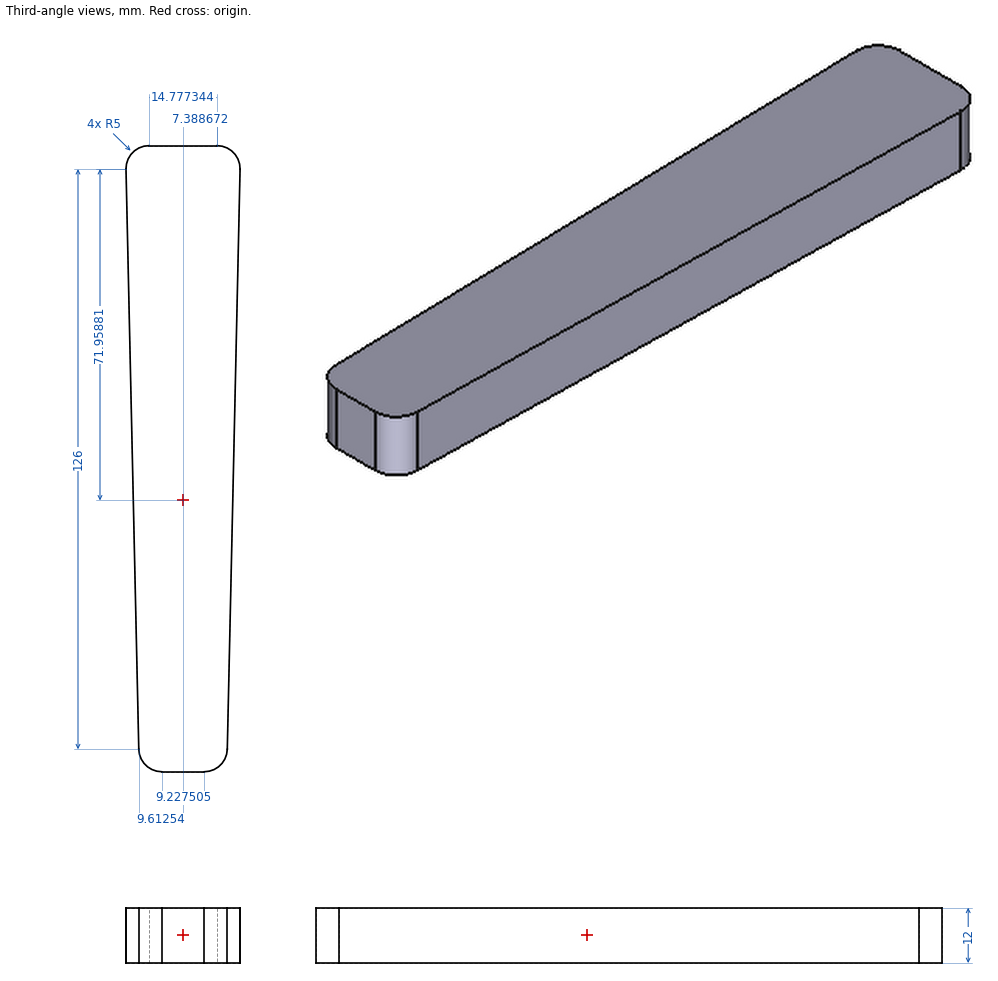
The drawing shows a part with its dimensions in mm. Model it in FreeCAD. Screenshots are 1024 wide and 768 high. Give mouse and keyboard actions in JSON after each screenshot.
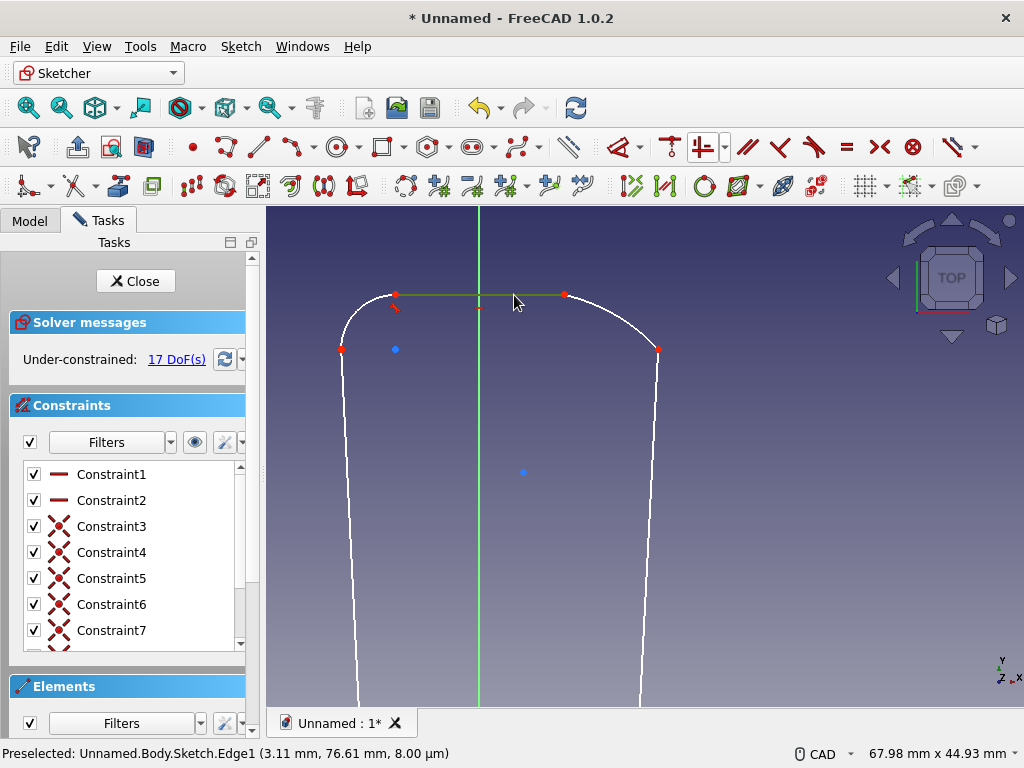
{"action": "left_click", "coordinate": [634, 327]}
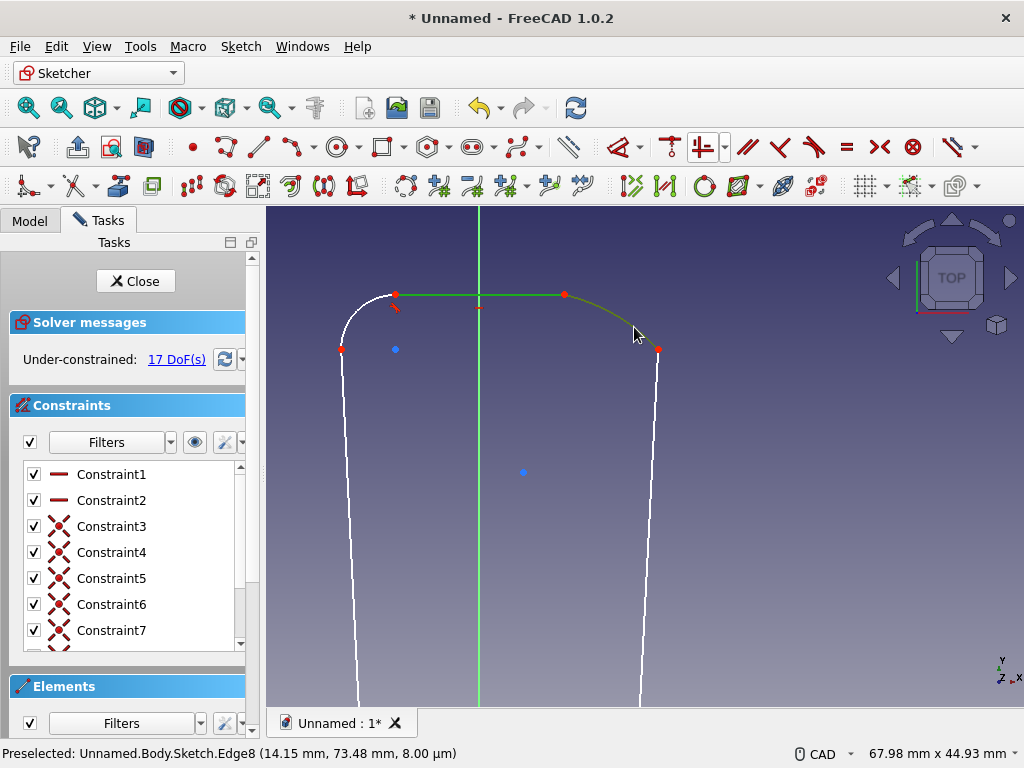
{"action": "key", "text": "t"}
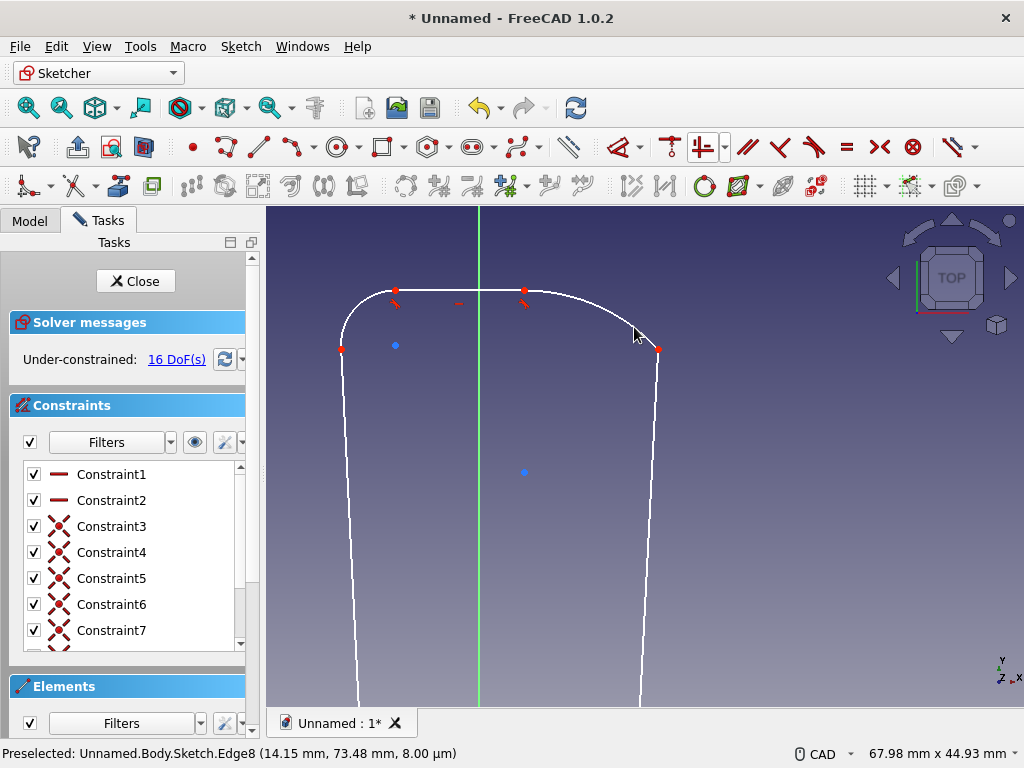
{"action": "scroll", "coordinate": [601, 307], "scroll_direction": "down", "scroll_amount": 8}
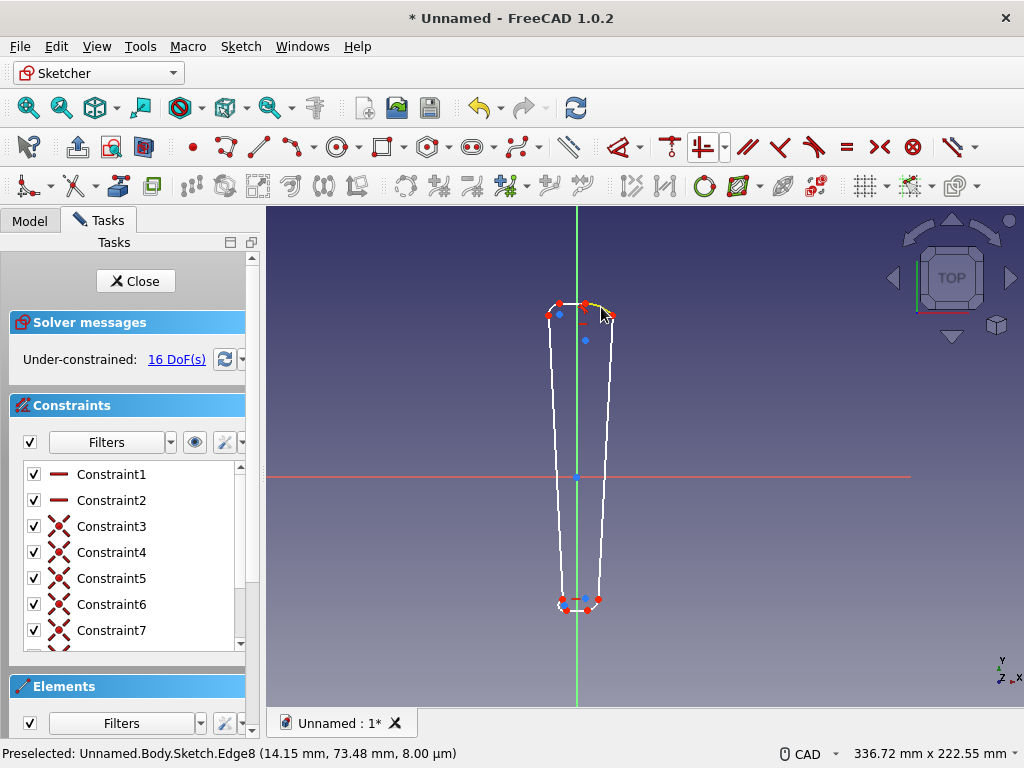
{"action": "left_click", "coordinate": [552, 373]}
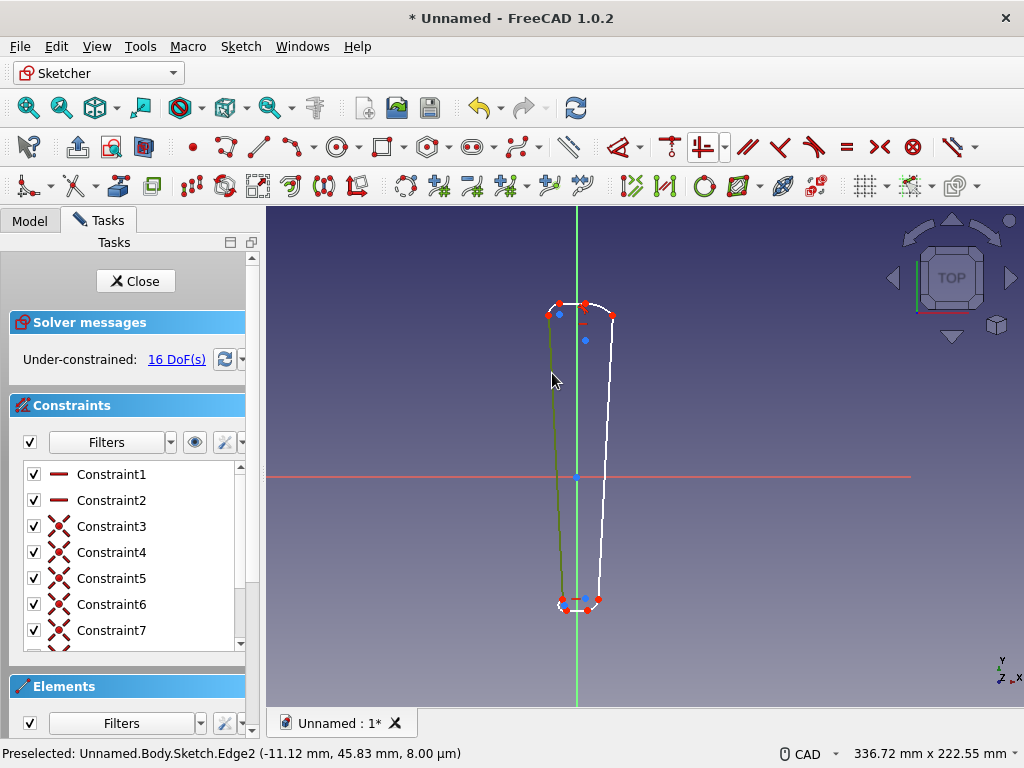
{"action": "scroll", "coordinate": [552, 307], "scroll_direction": "up", "scroll_amount": 3}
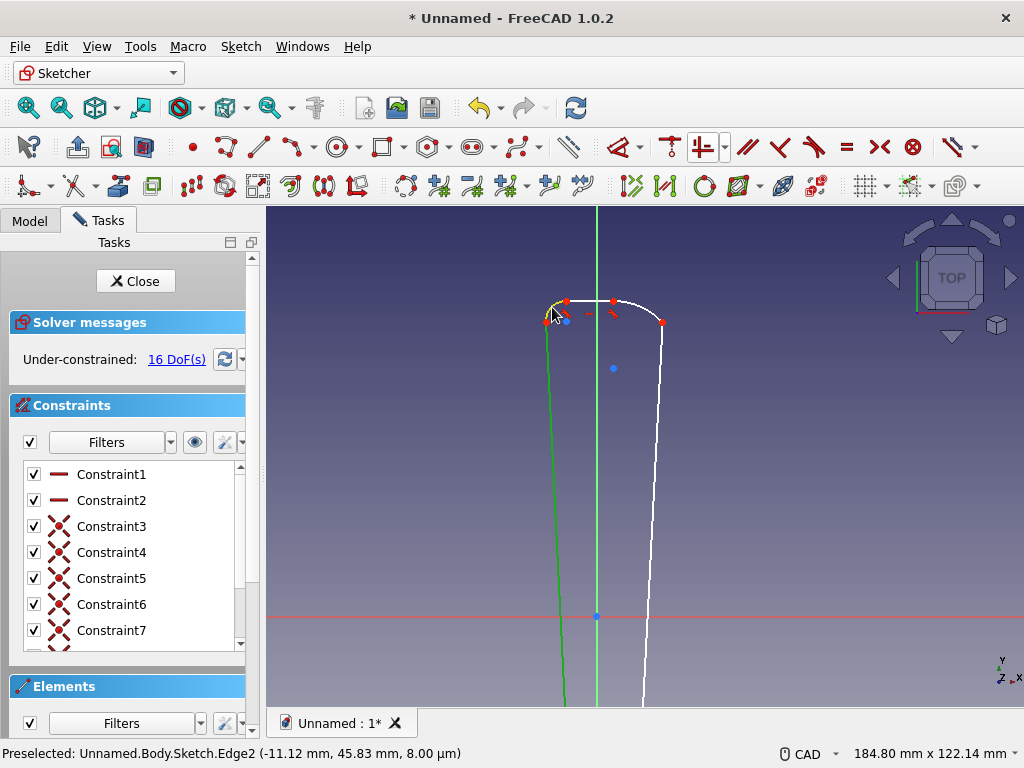
{"action": "left_click", "coordinate": [551, 308]}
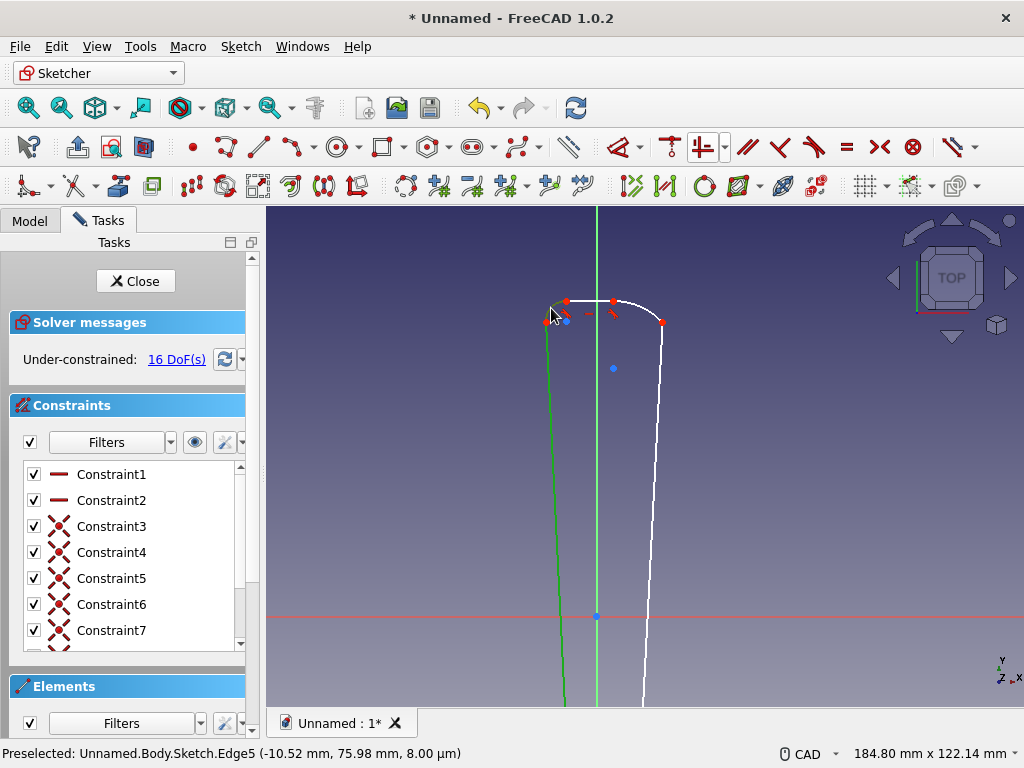
{"action": "left_click", "coordinate": [814, 148]}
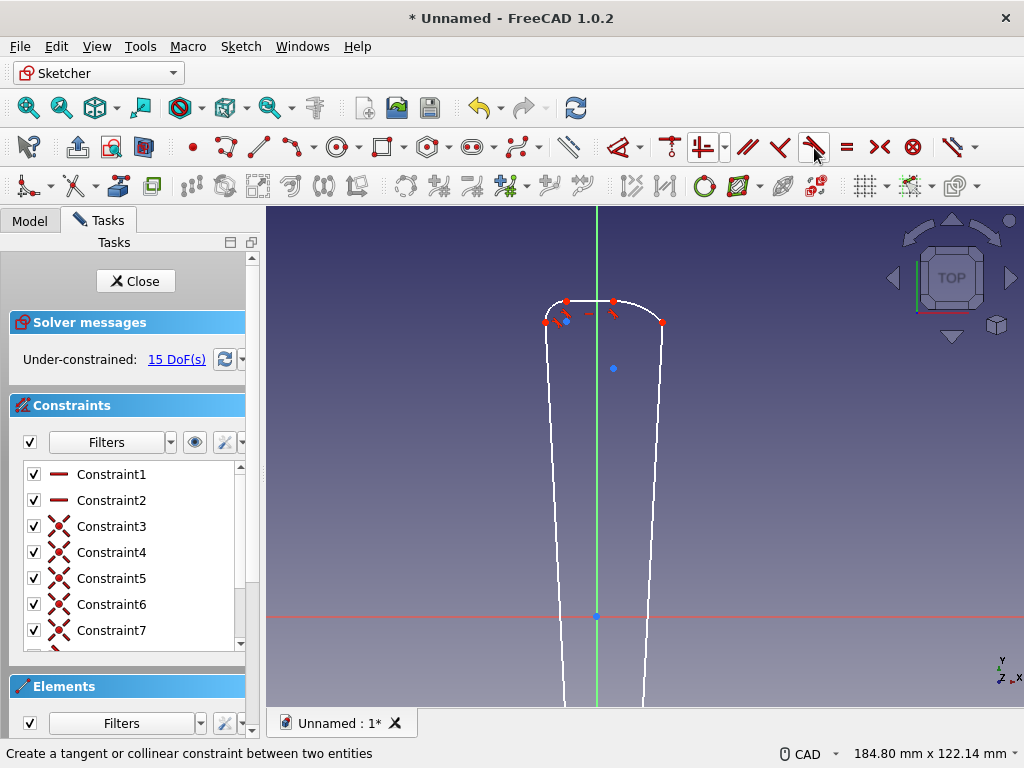
{"action": "left_click", "coordinate": [553, 478]}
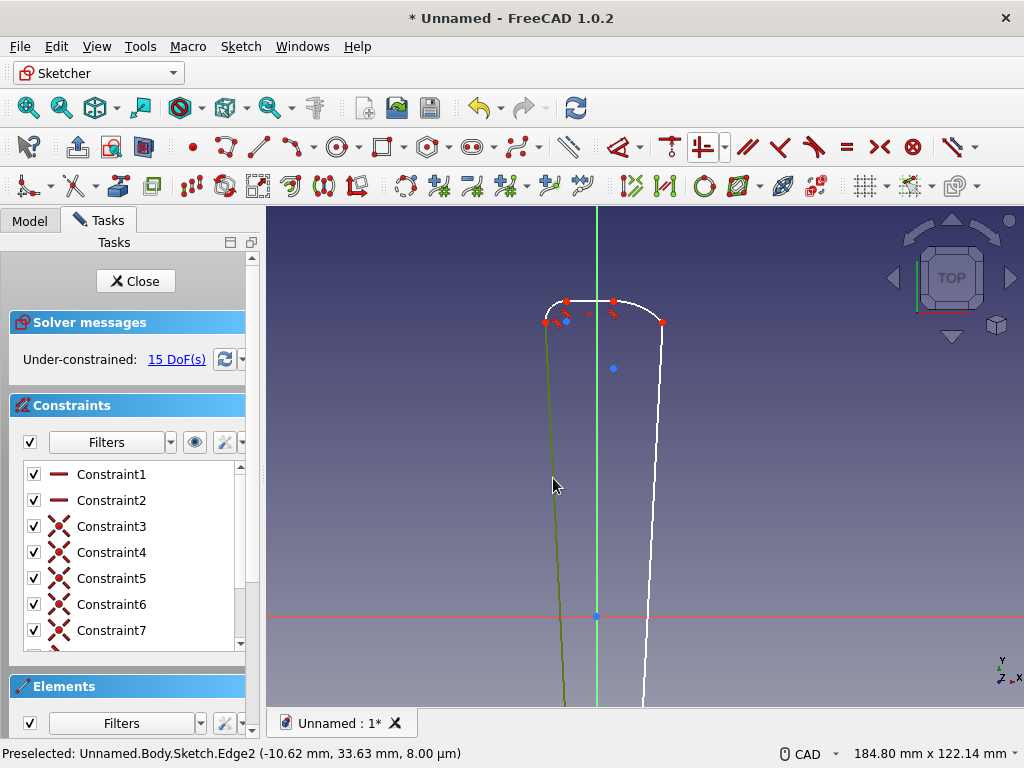
{"action": "scroll", "coordinate": [552, 307], "scroll_direction": "down", "scroll_amount": 3}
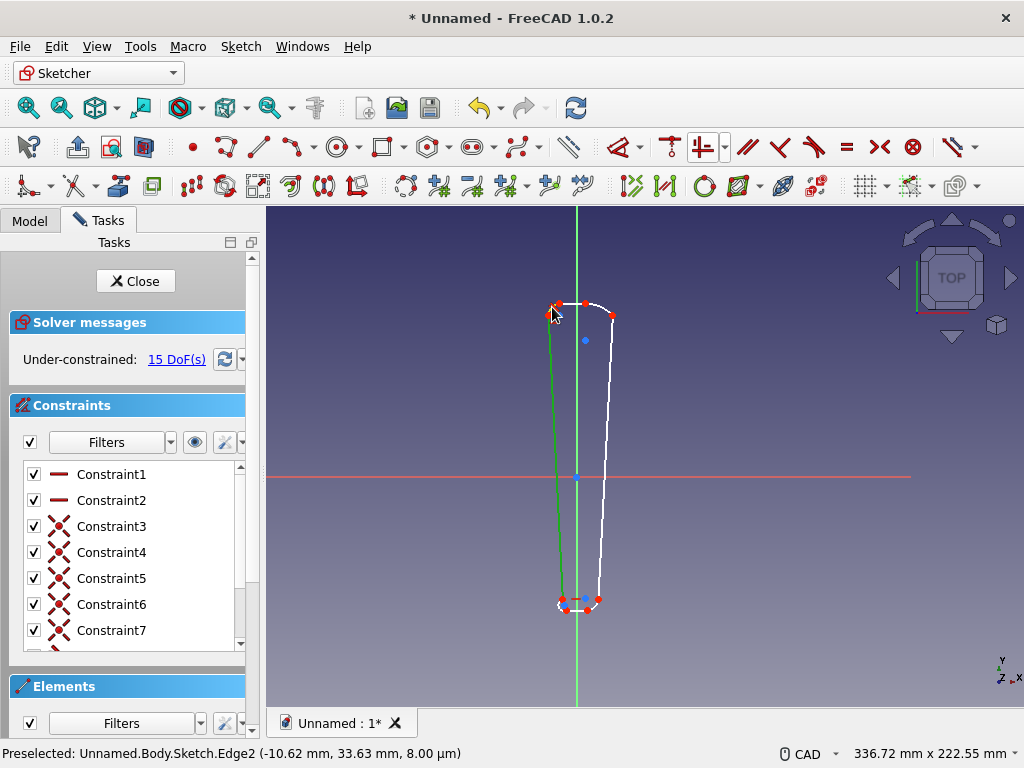
{"action": "scroll", "coordinate": [559, 603], "scroll_direction": "up", "scroll_amount": 5}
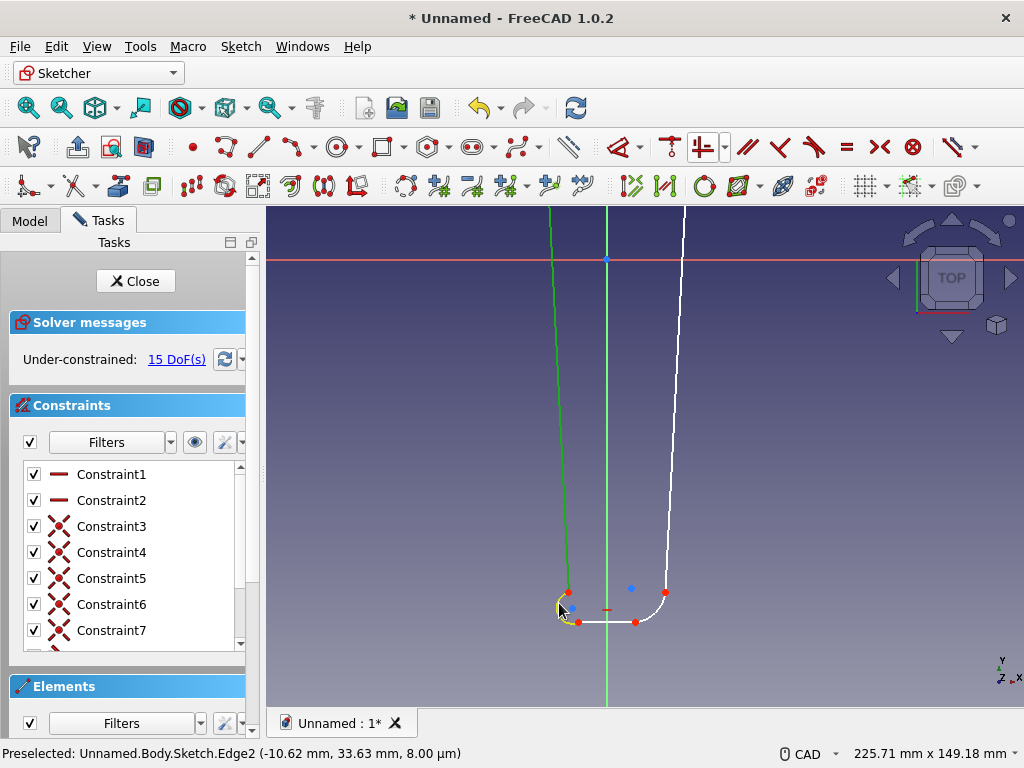
{"action": "left_click", "coordinate": [558, 603]}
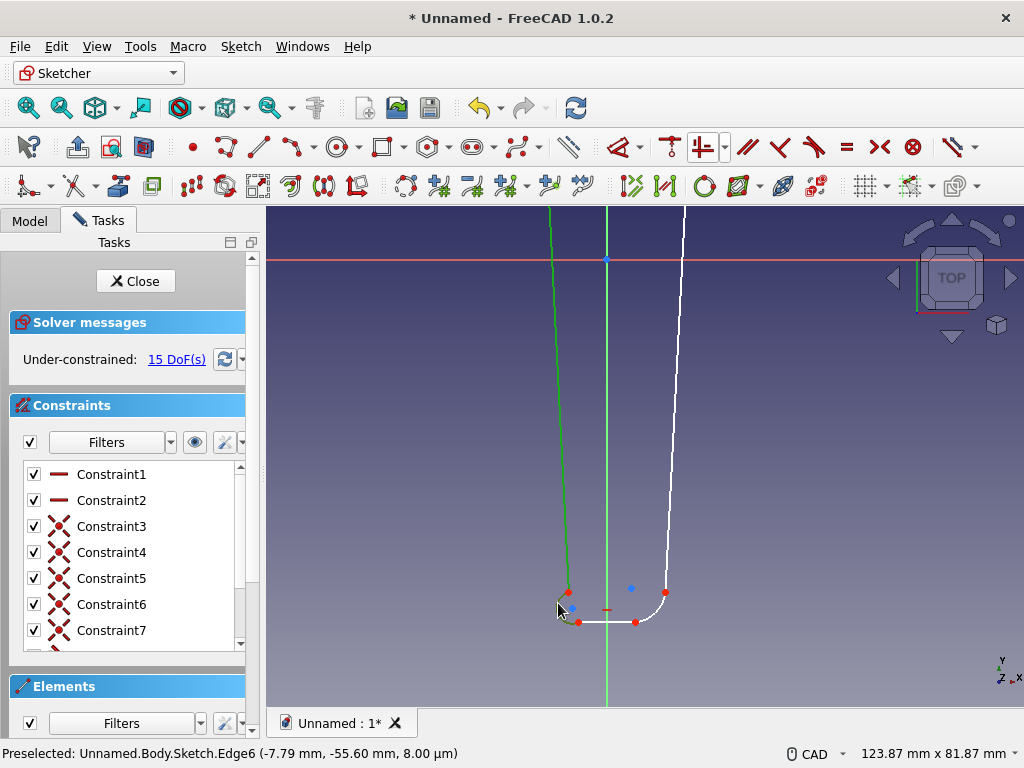
{"action": "key", "text": "t"}